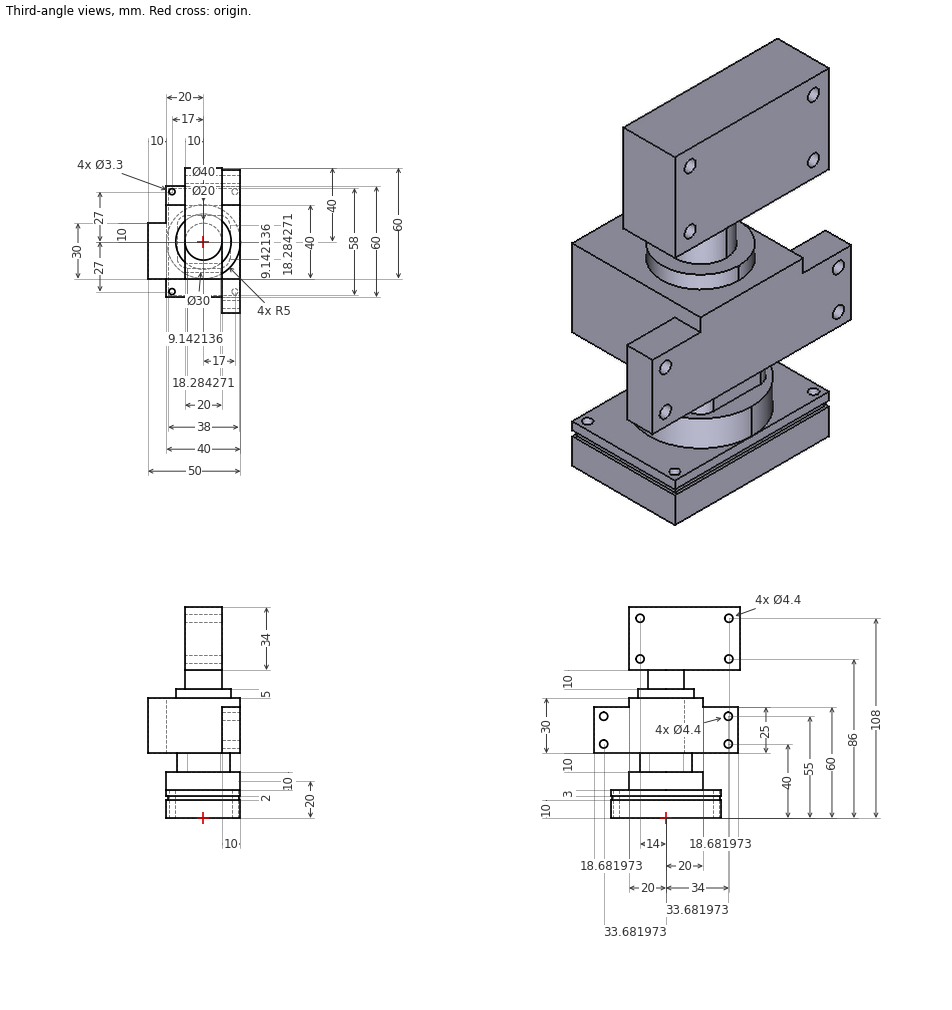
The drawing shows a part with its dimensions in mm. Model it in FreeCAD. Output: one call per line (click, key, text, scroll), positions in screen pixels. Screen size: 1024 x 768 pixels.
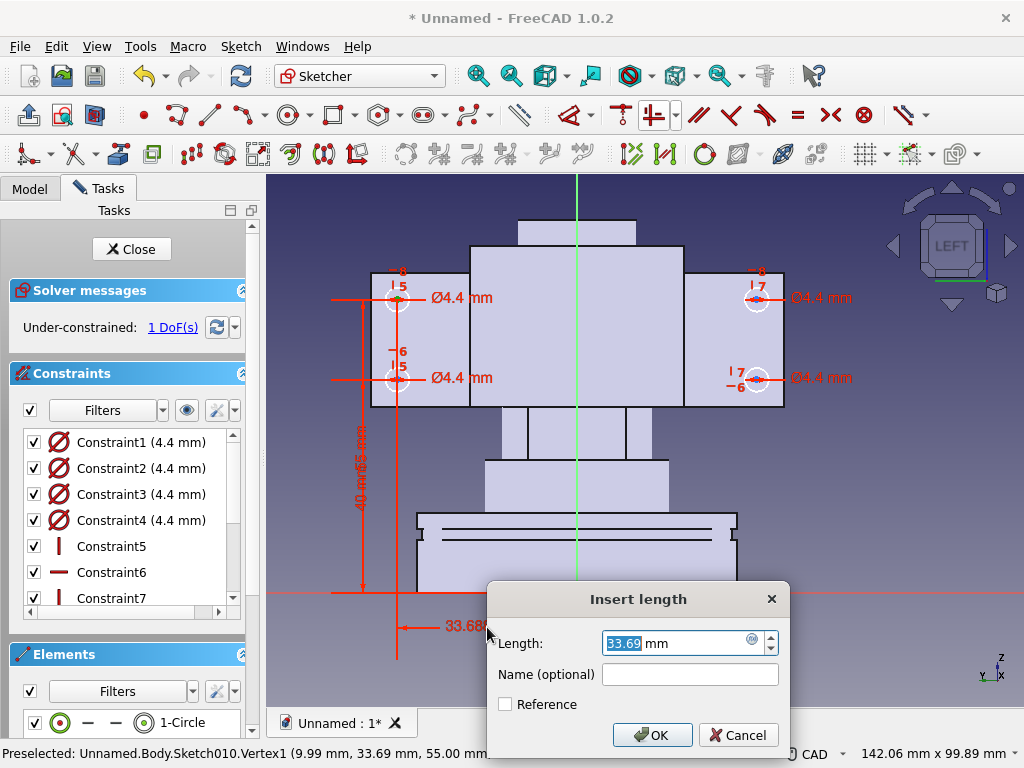
text(33.681973)
key(Return)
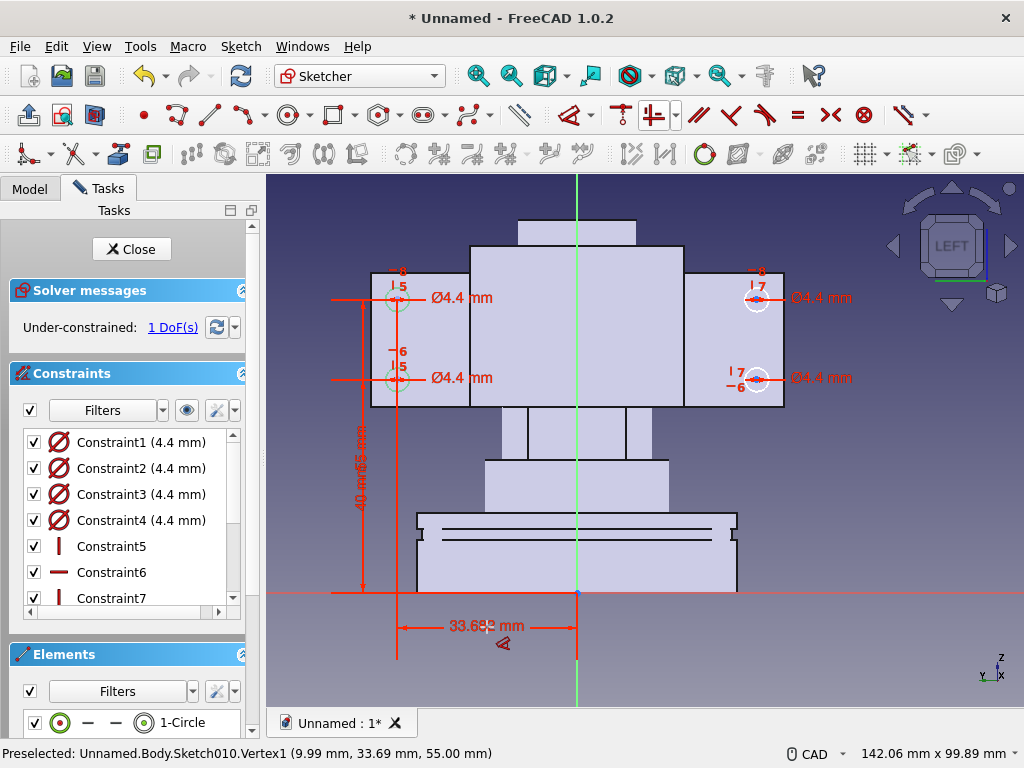
click(757, 380)
click(667, 627)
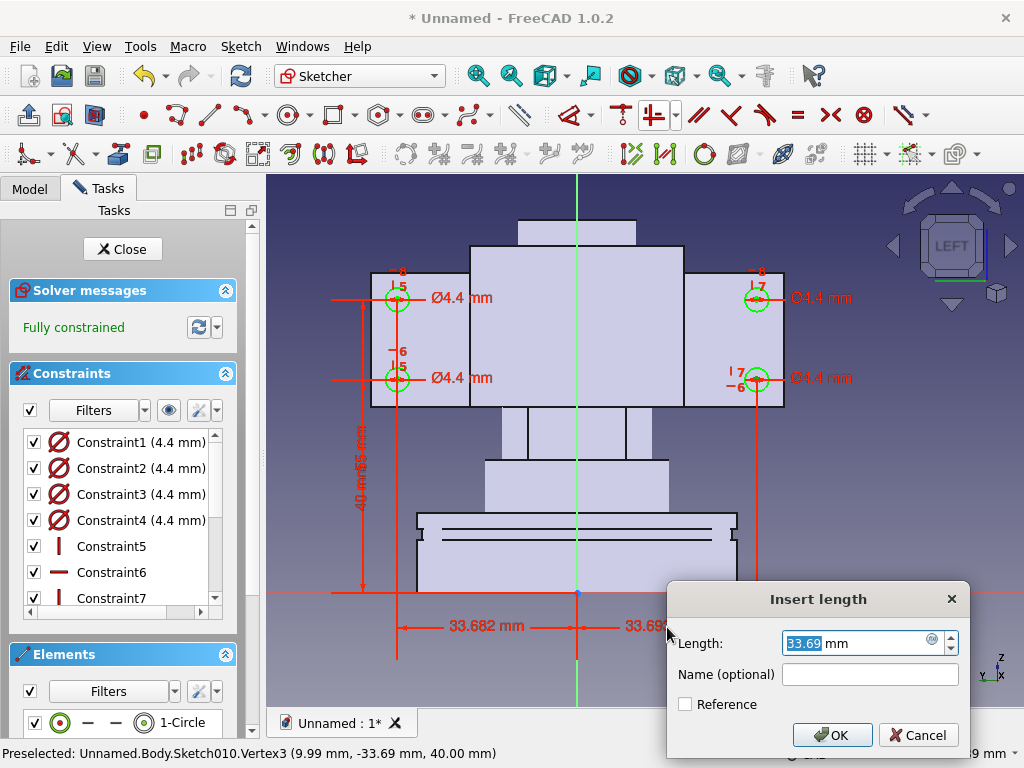
text(33.681973)
key(Return)
key(Escape)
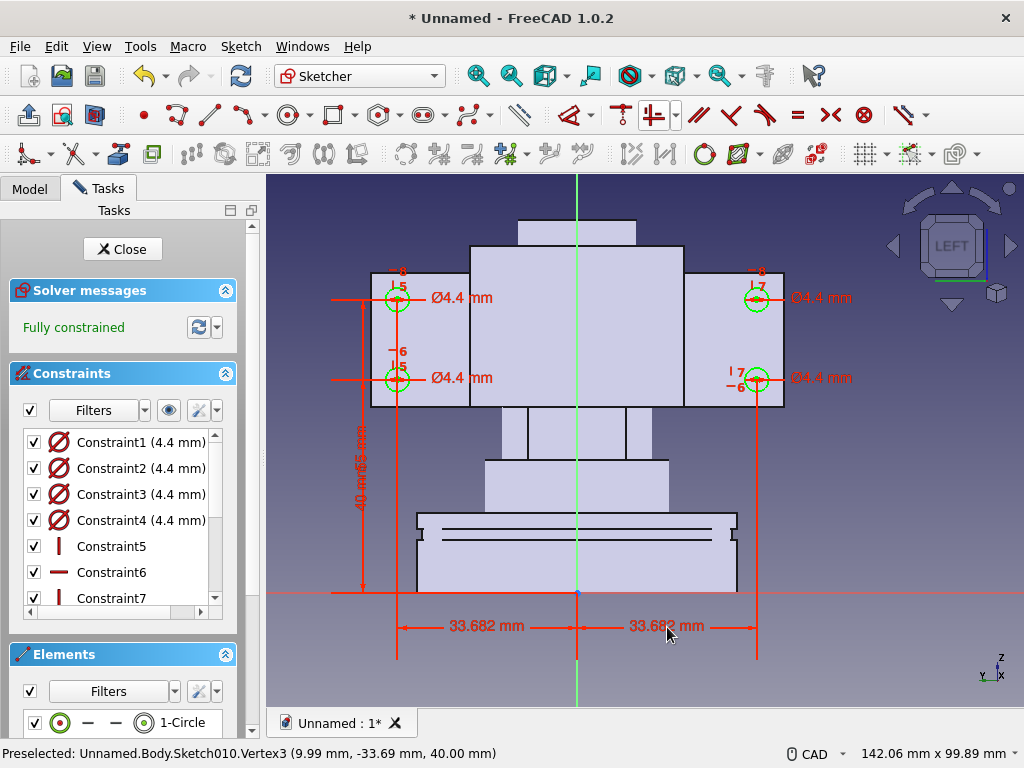
click(123, 249)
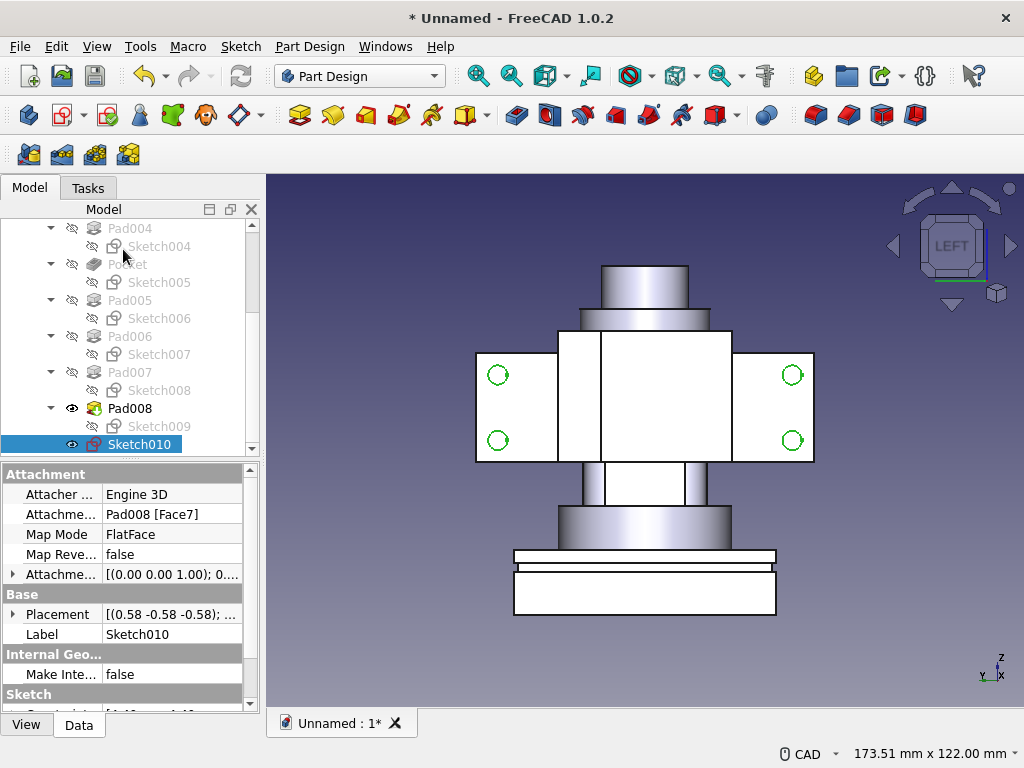
click(517, 116)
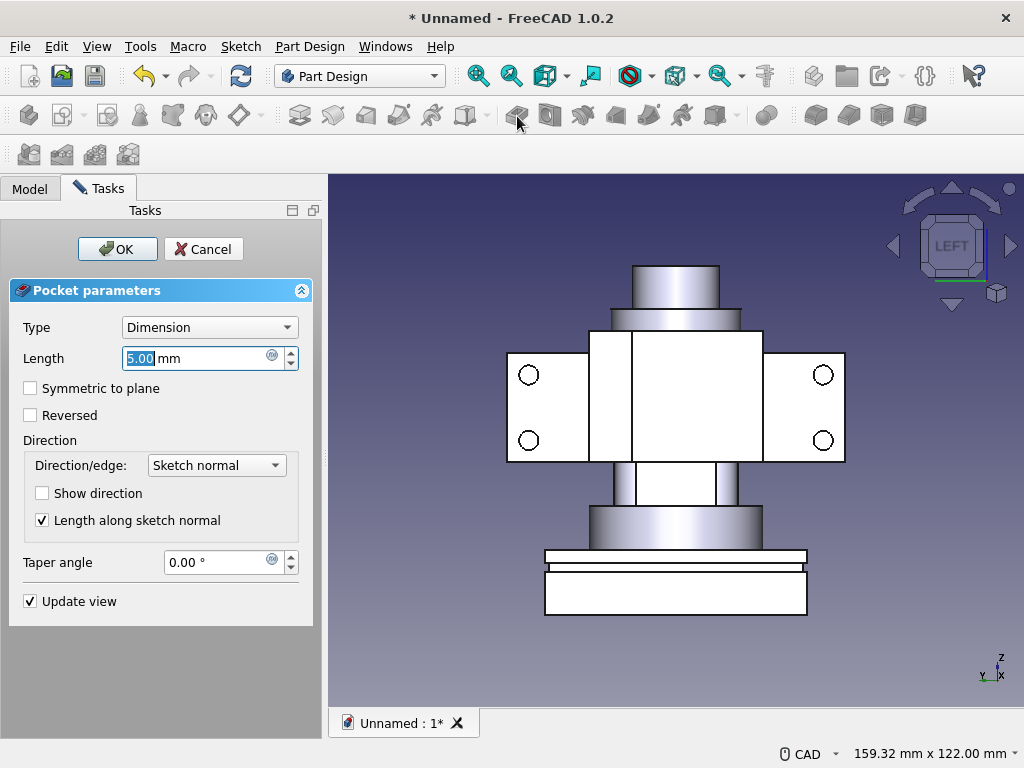
text(10)
key(Tab)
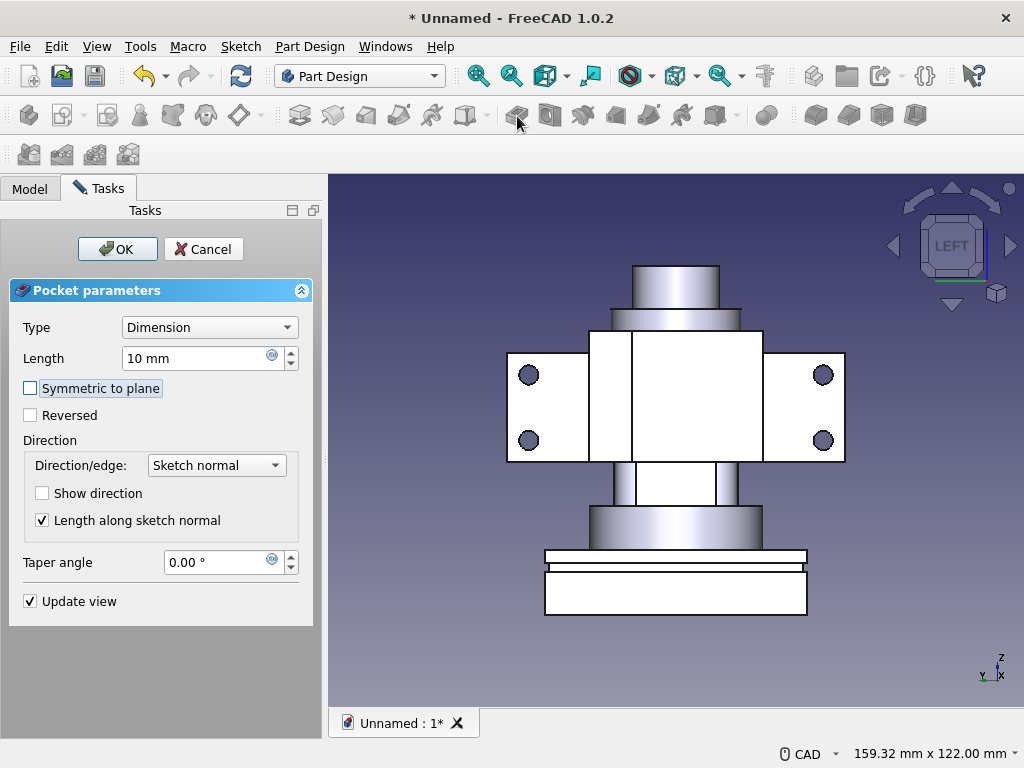
click(118, 249)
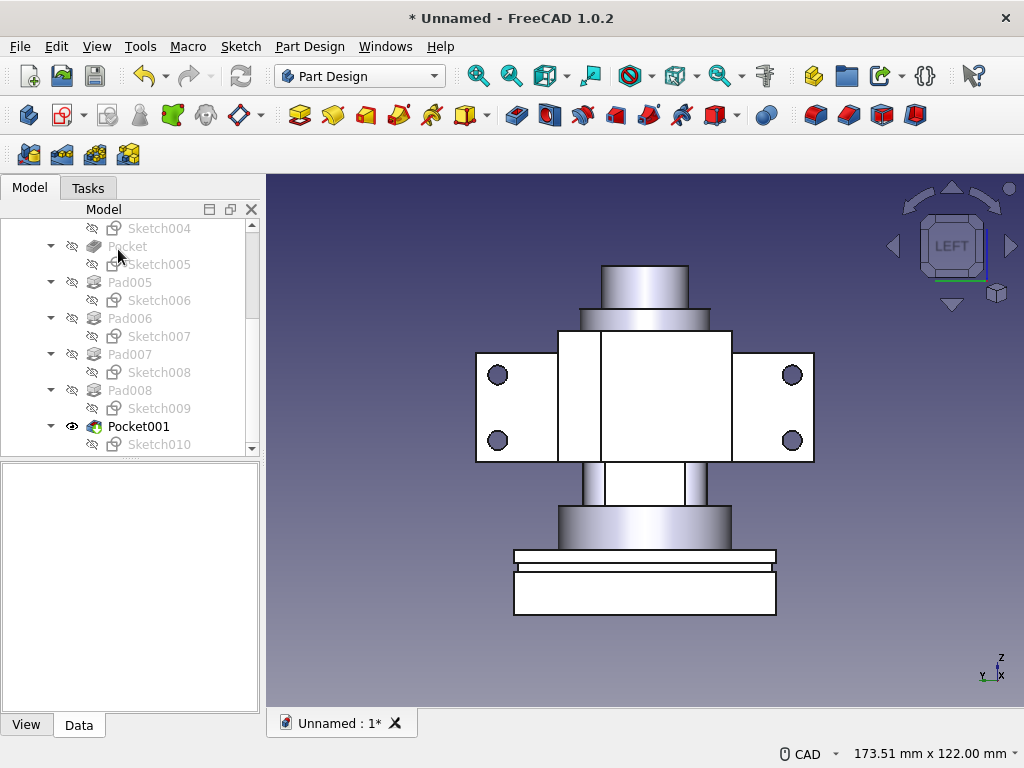
key(0)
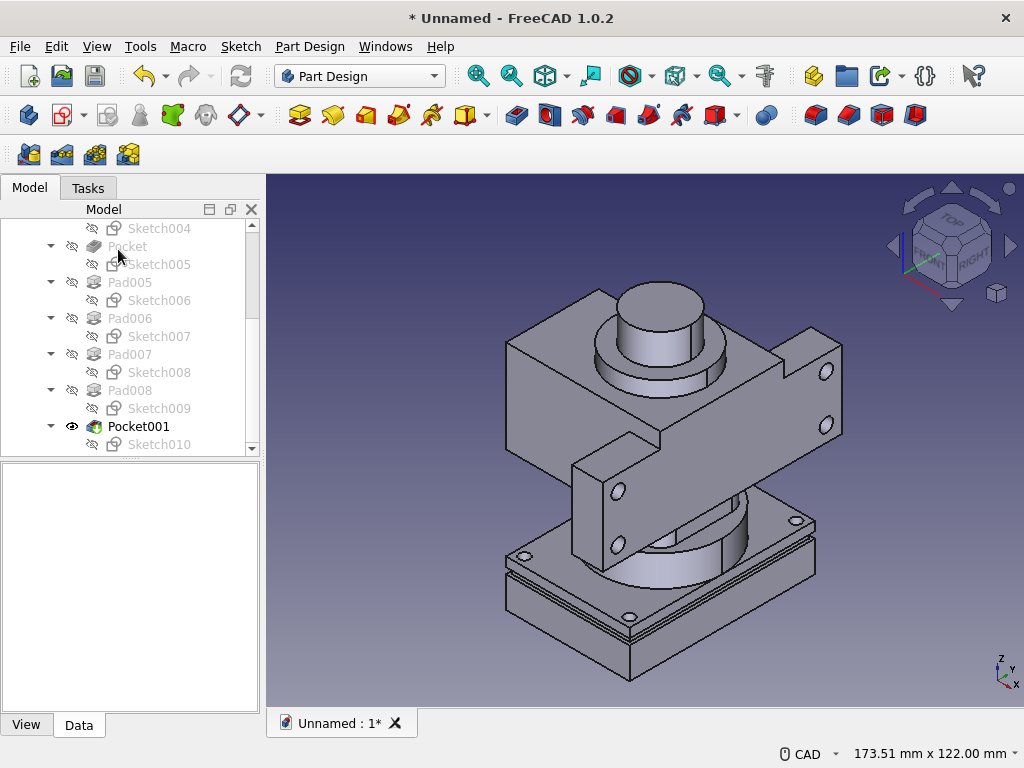
click(660, 306)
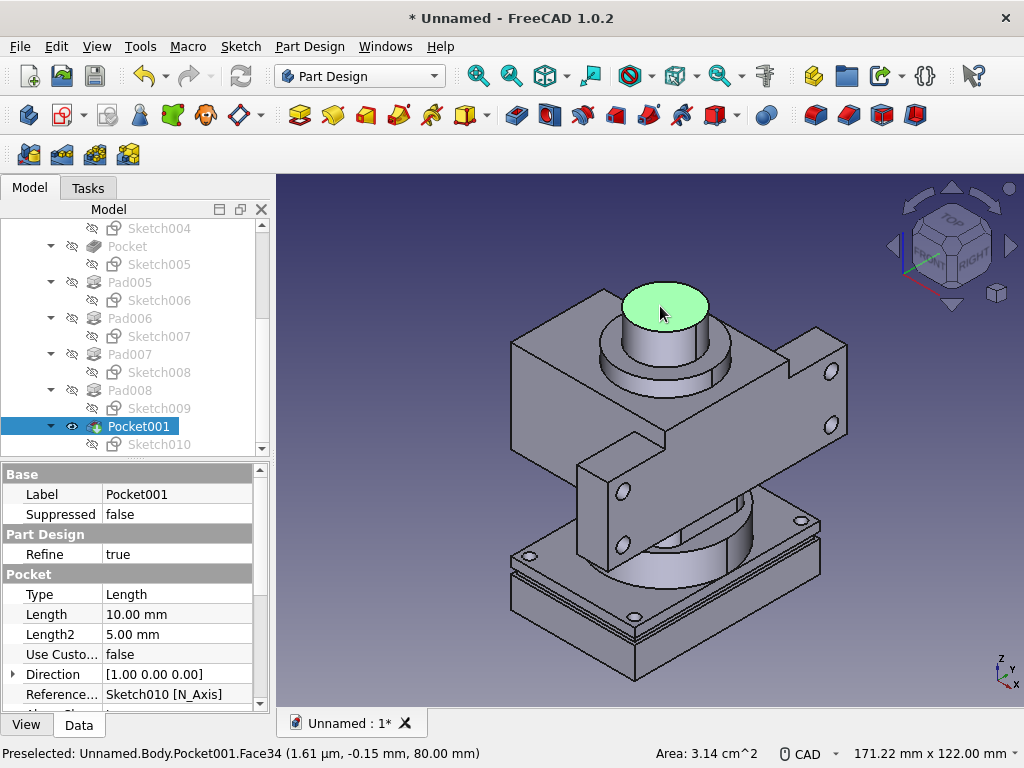
click(62, 116)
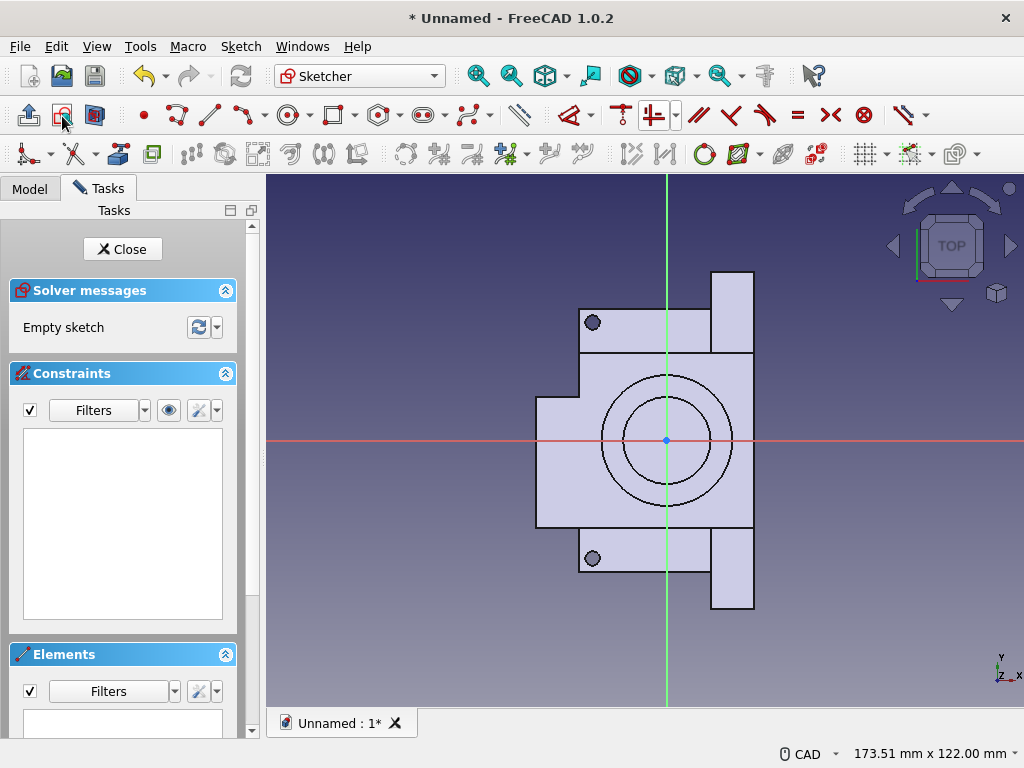
click(332, 116)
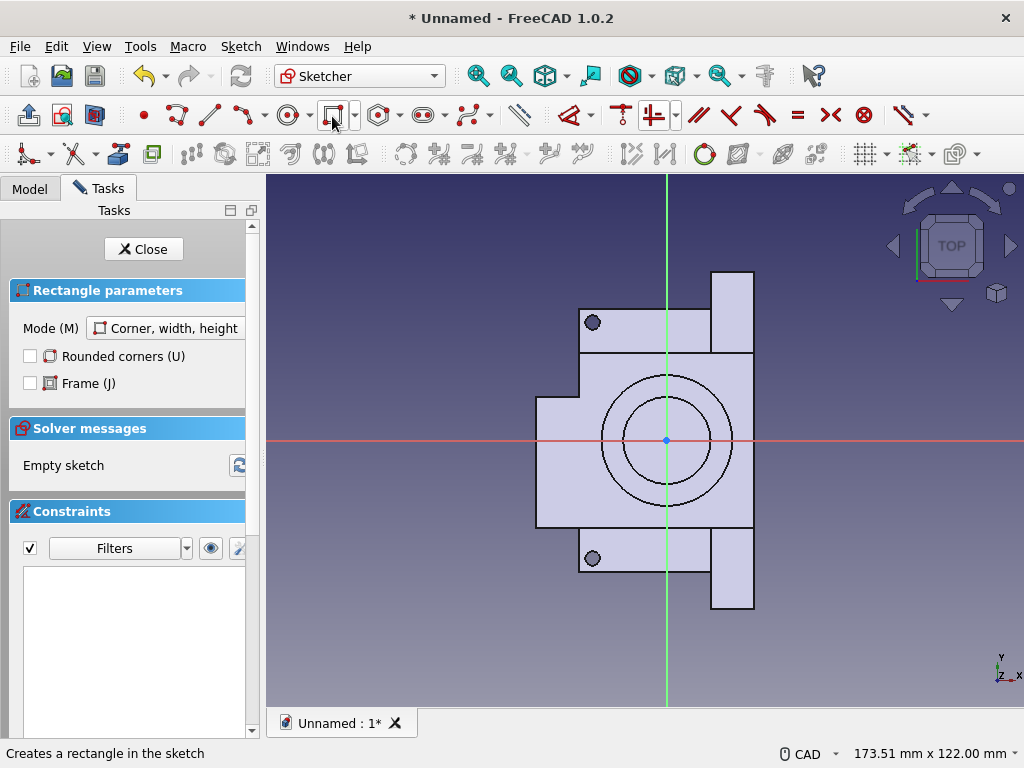
click(623, 266)
move(711, 528)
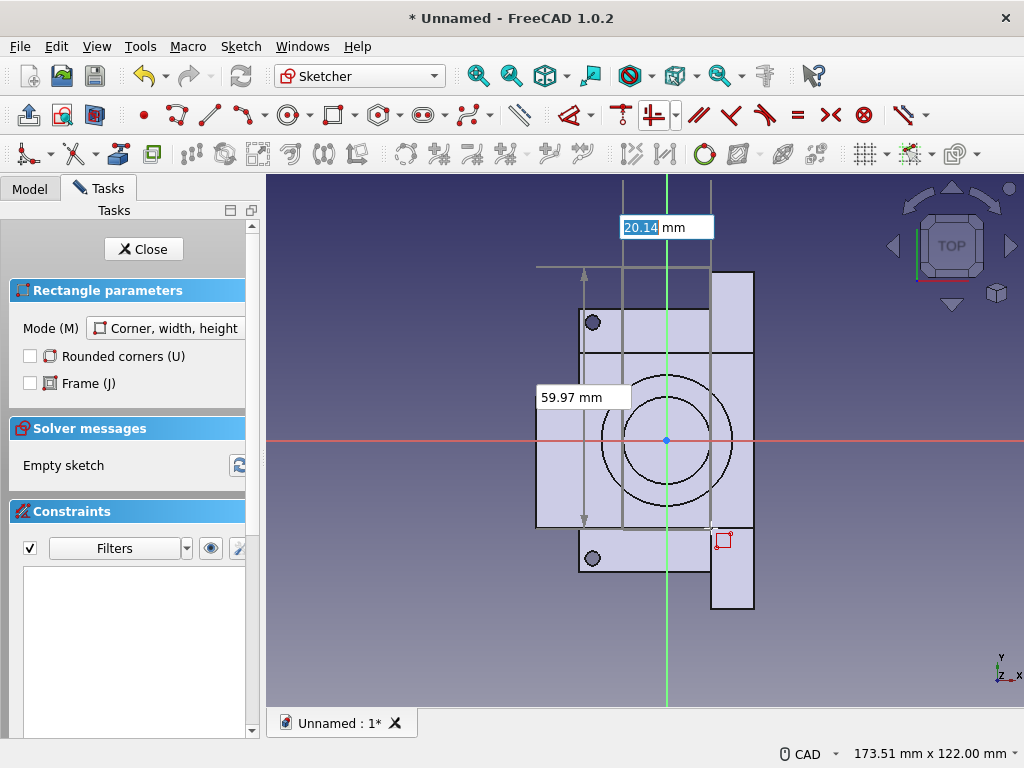
text(20)
key(Tab)
text(60)
key(Return)
key(Escape)